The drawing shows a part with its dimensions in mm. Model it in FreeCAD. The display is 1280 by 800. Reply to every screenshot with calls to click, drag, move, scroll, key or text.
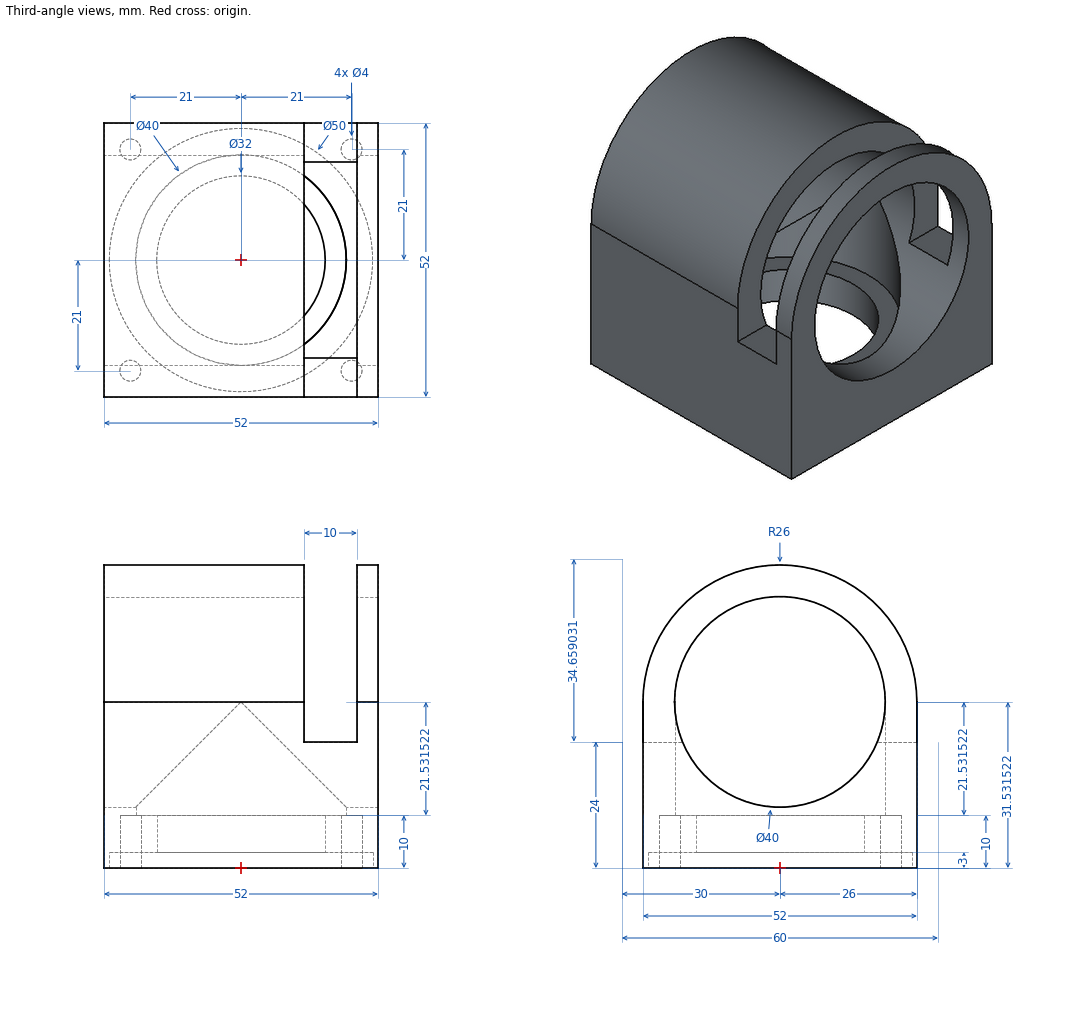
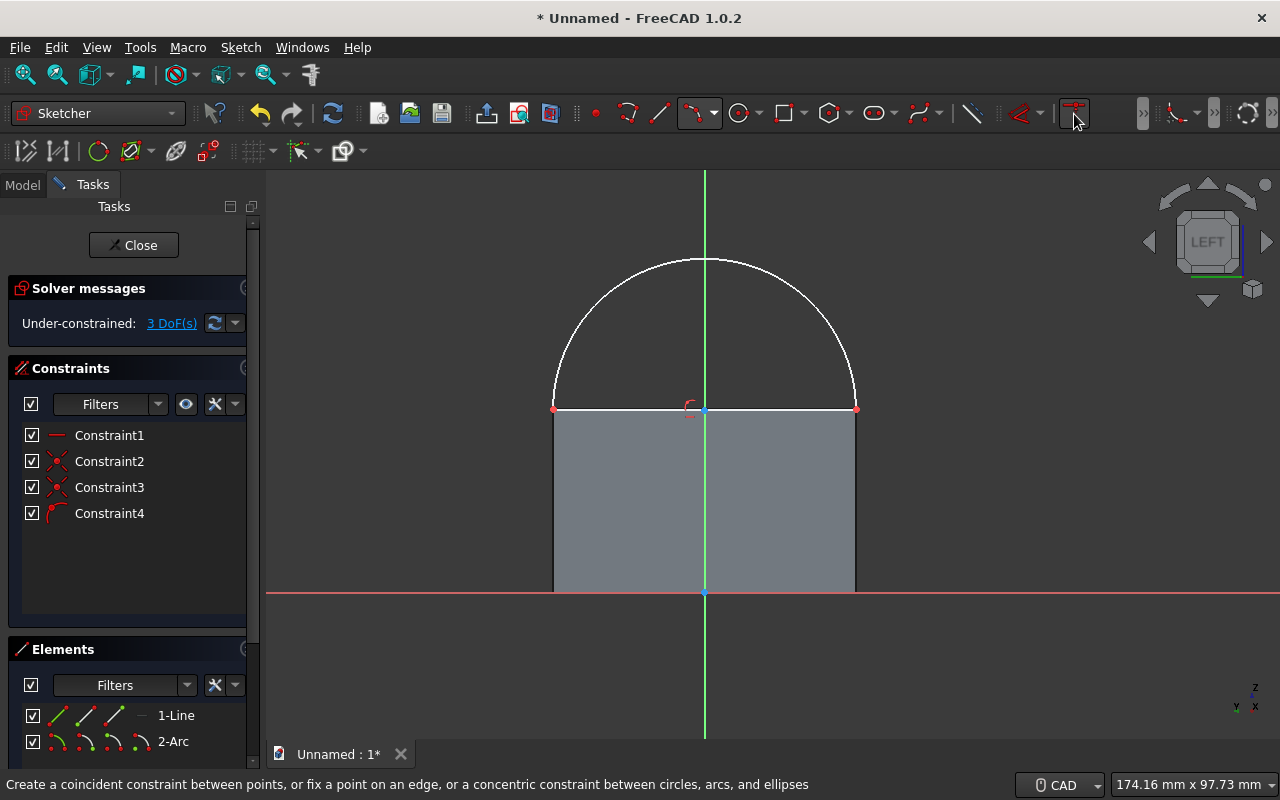
click(1020, 114)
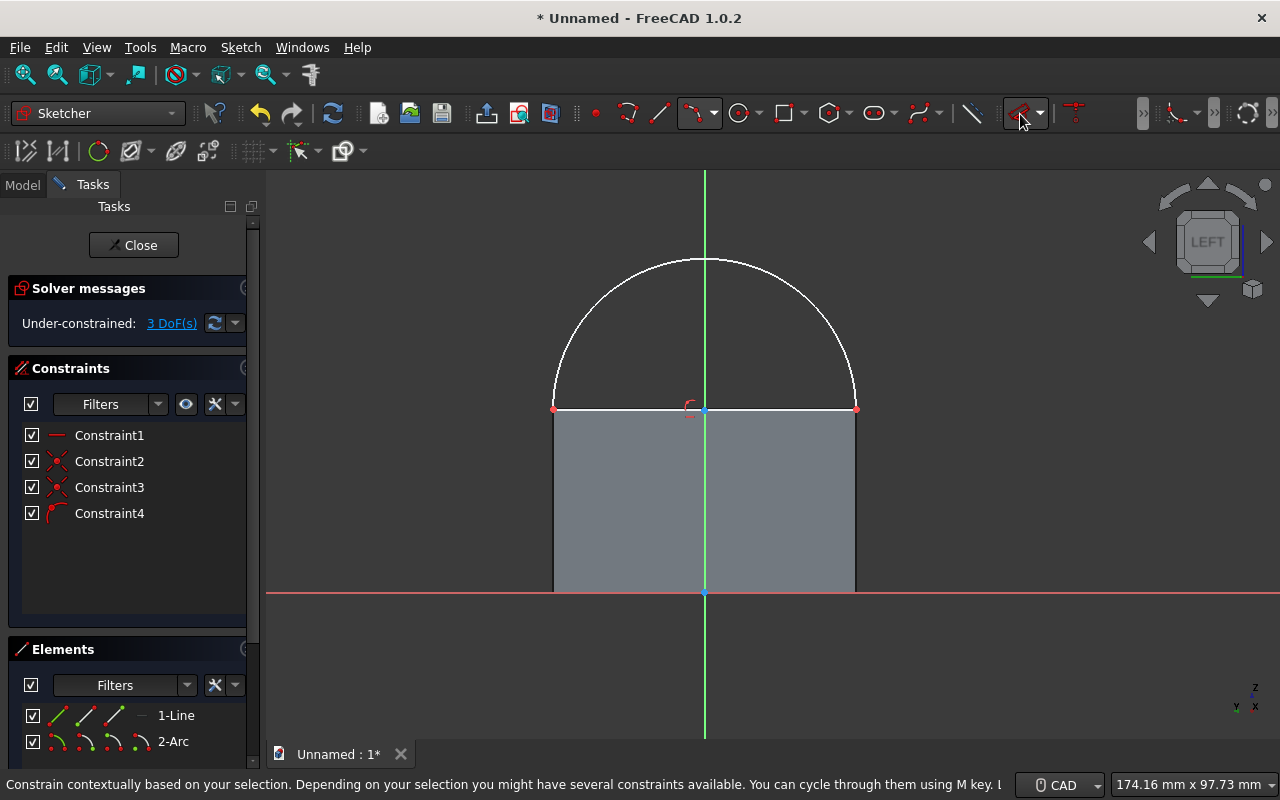
click(793, 288)
click(812, 262)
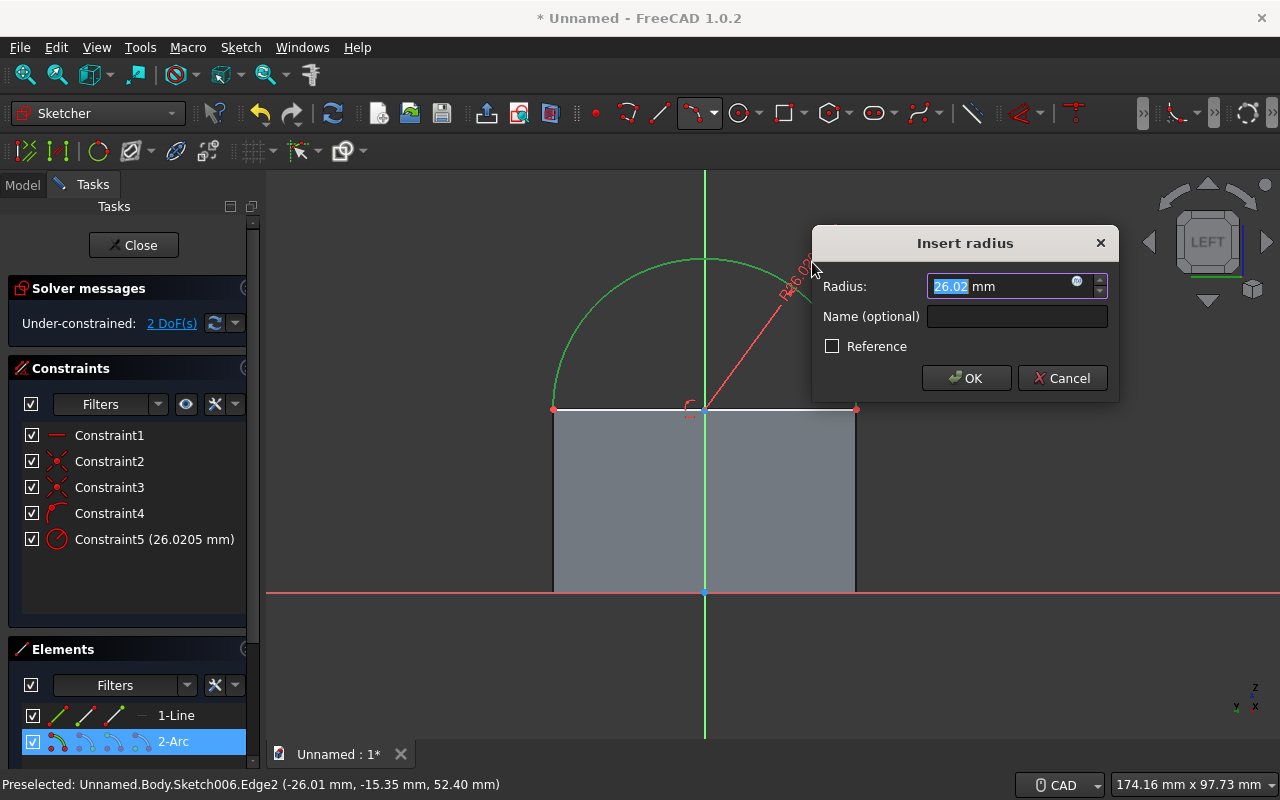
text(26)
key(Return)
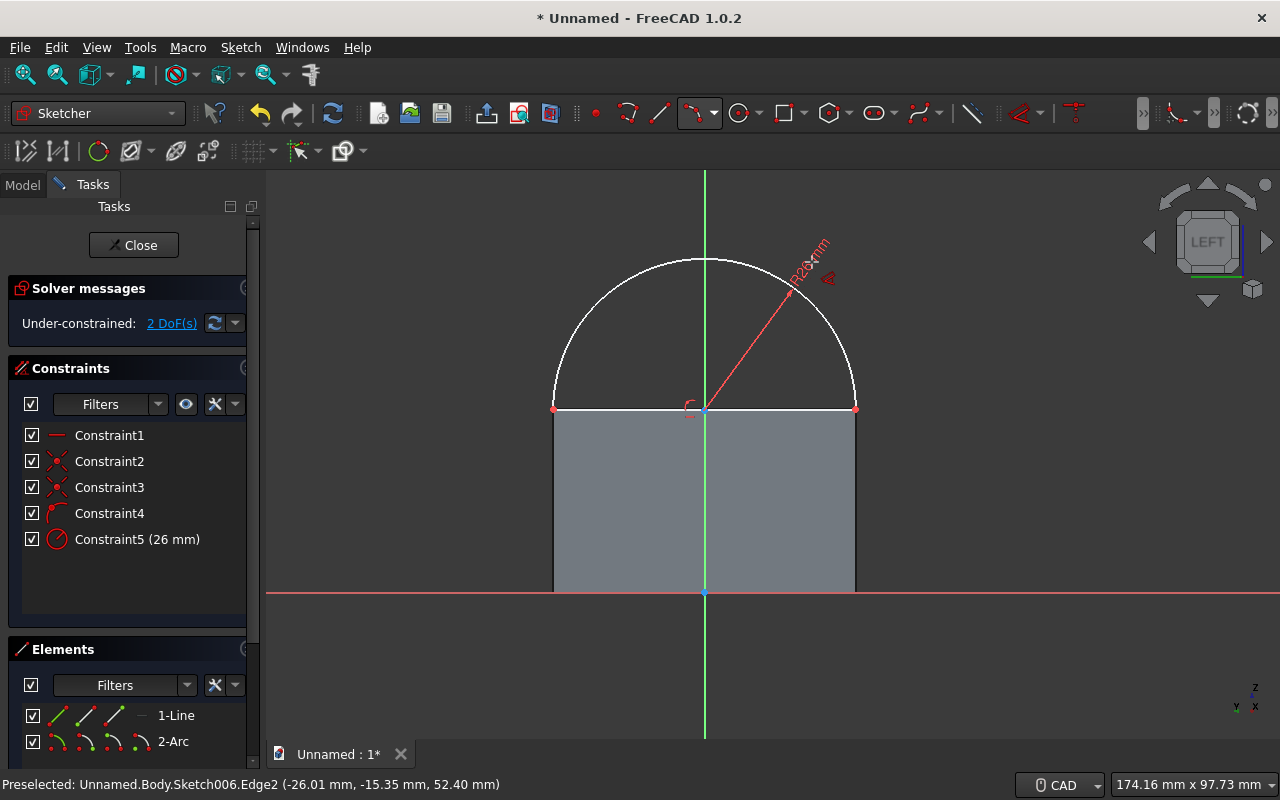
click(553, 410)
click(519, 501)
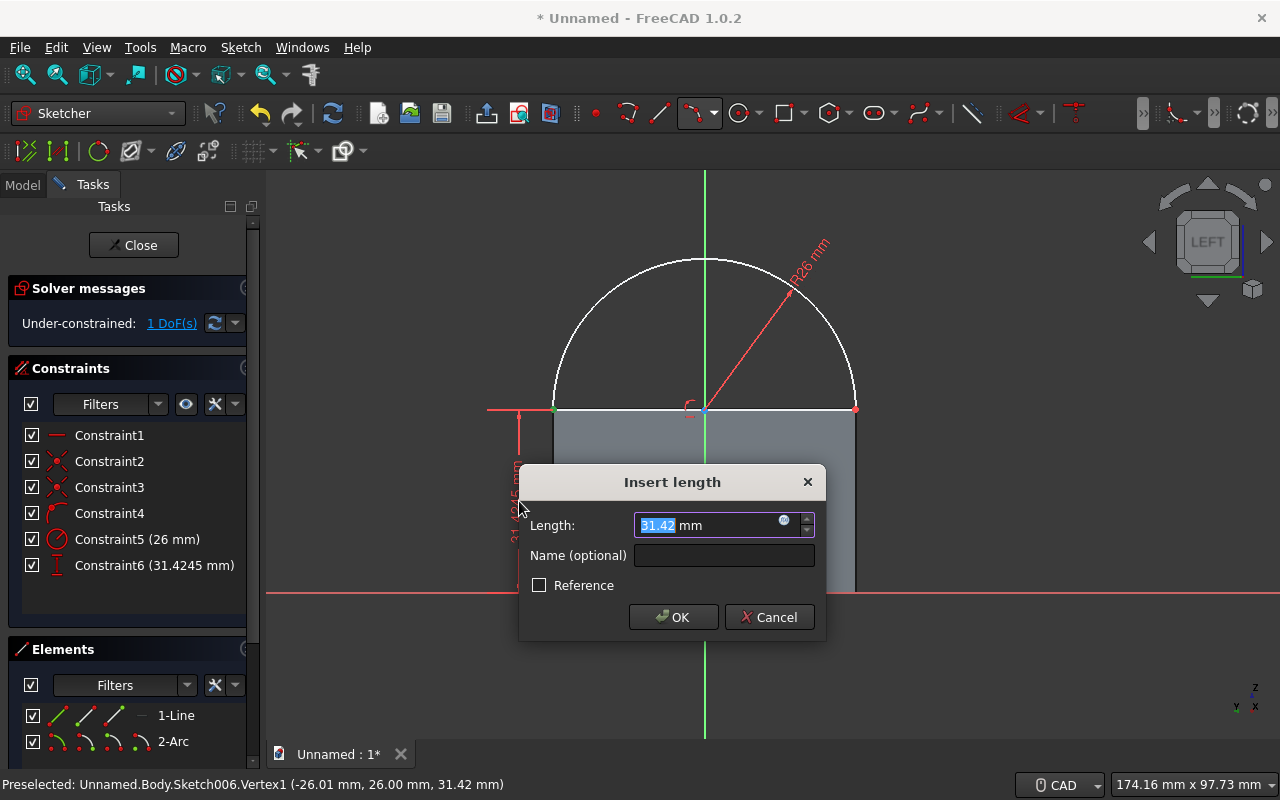
text(31.531522)
key(Return)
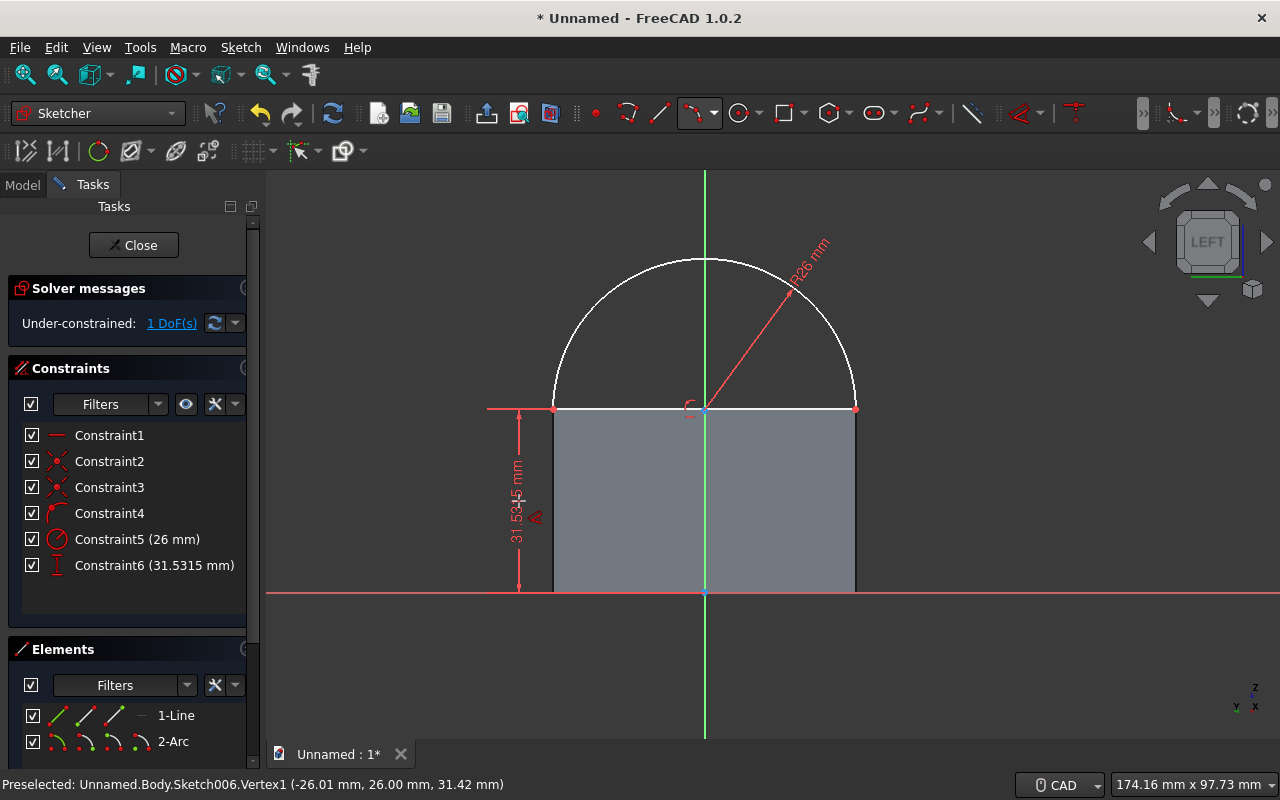
click(705, 410)
click(739, 502)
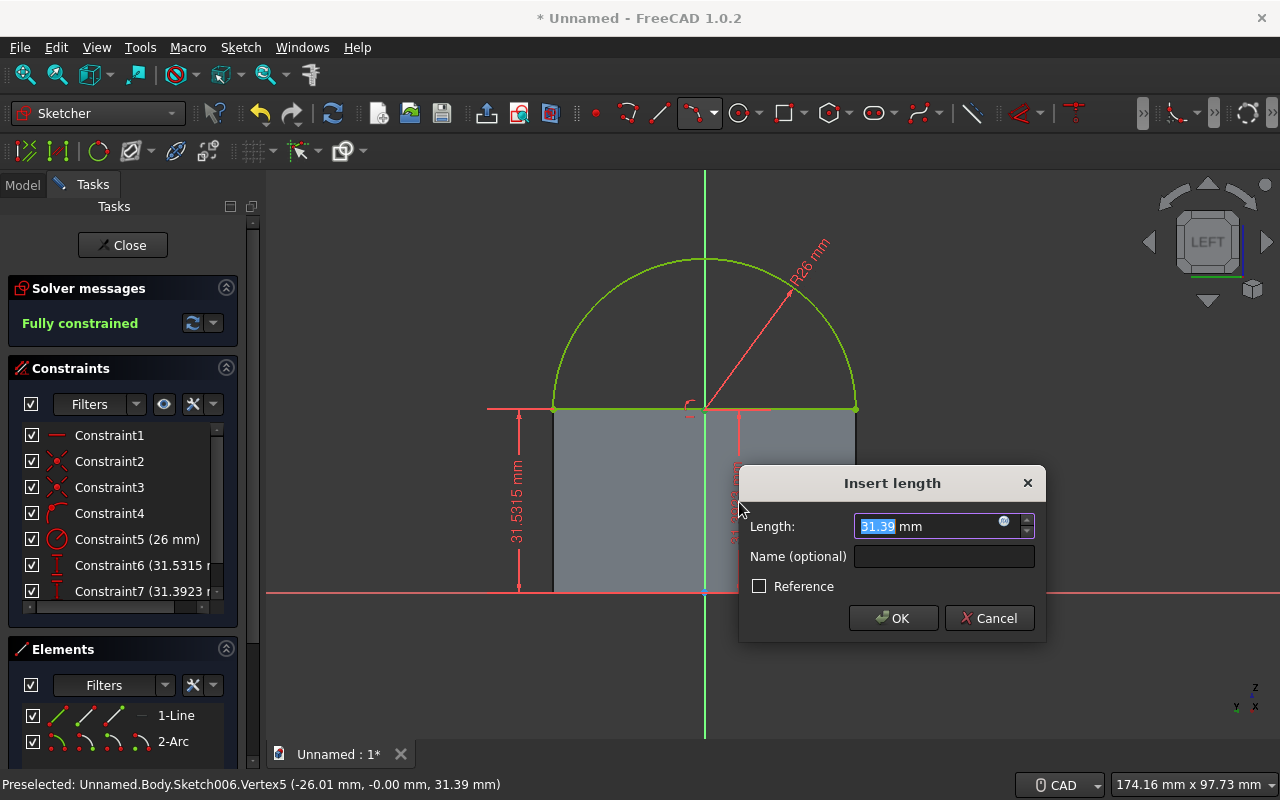
text(31.531522)
key(Return)
key(Escape)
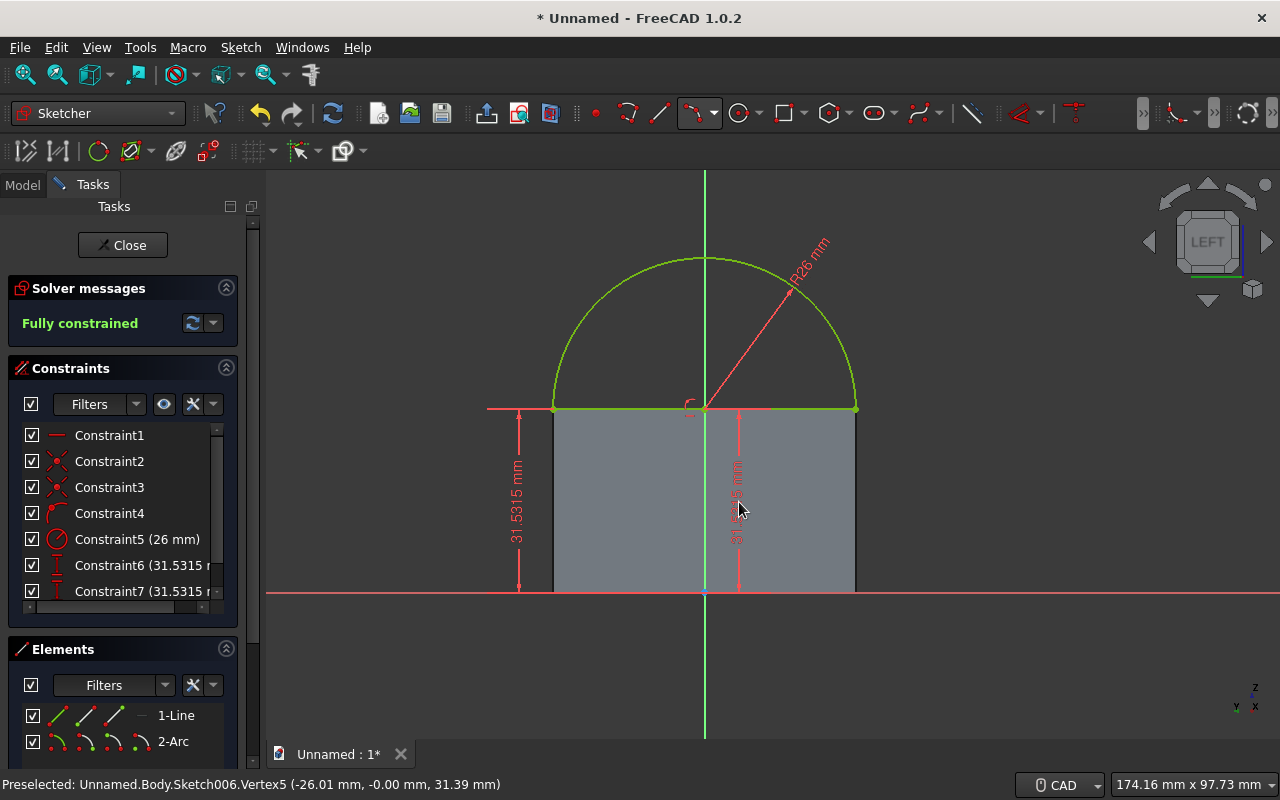
click(123, 245)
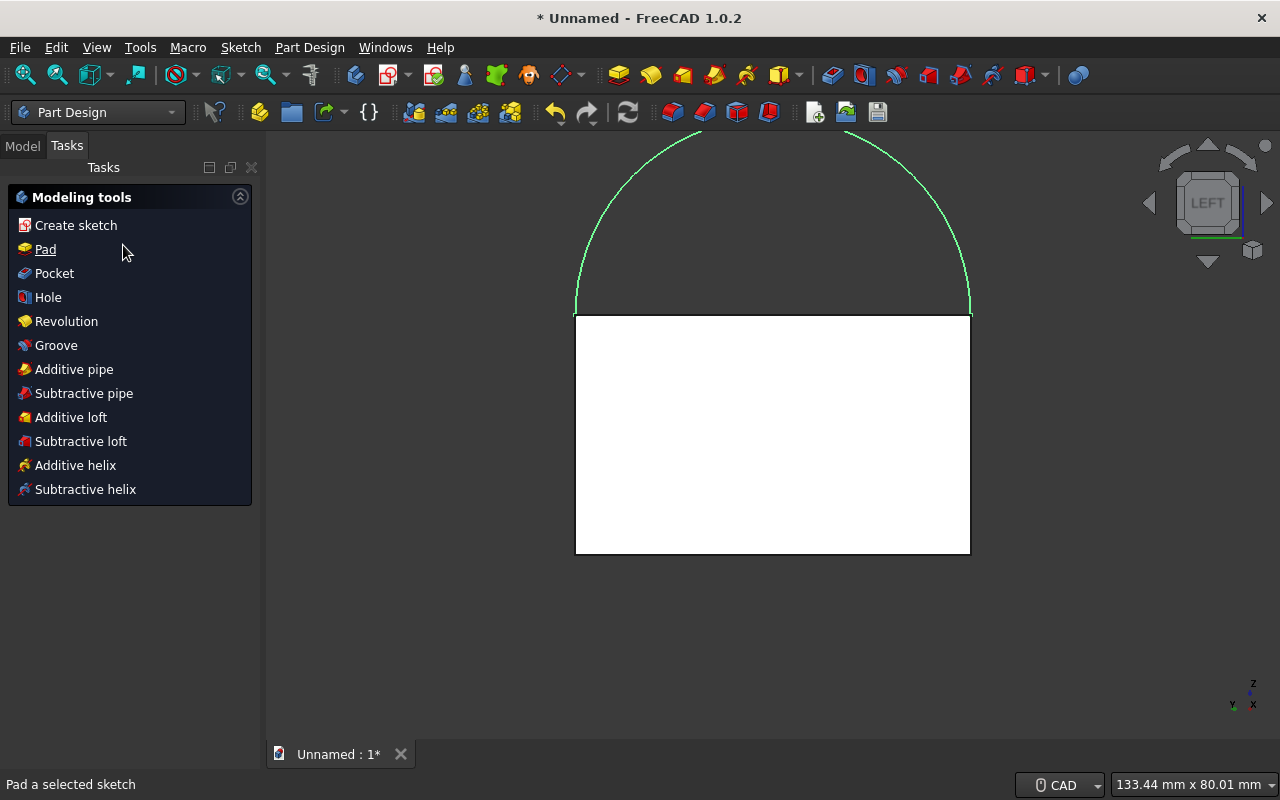
click(620, 76)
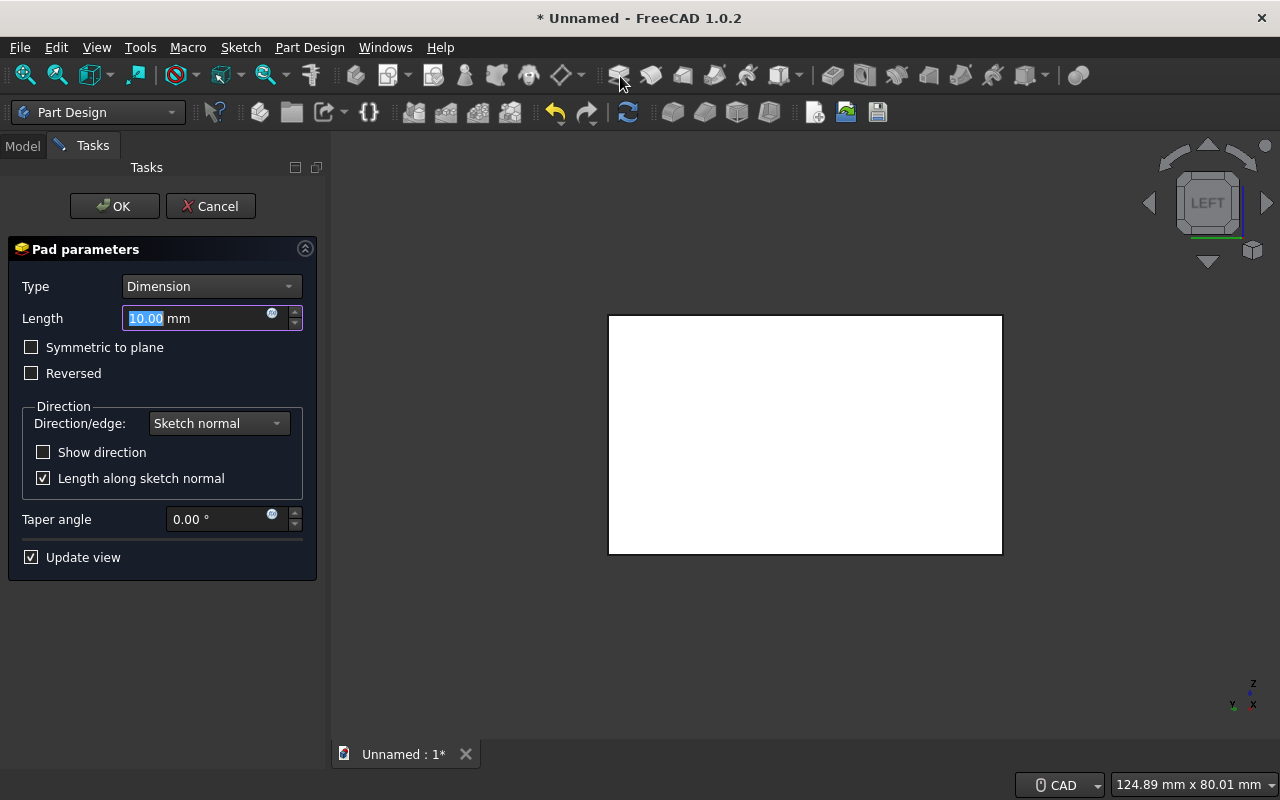
text(52)
key(Tab)